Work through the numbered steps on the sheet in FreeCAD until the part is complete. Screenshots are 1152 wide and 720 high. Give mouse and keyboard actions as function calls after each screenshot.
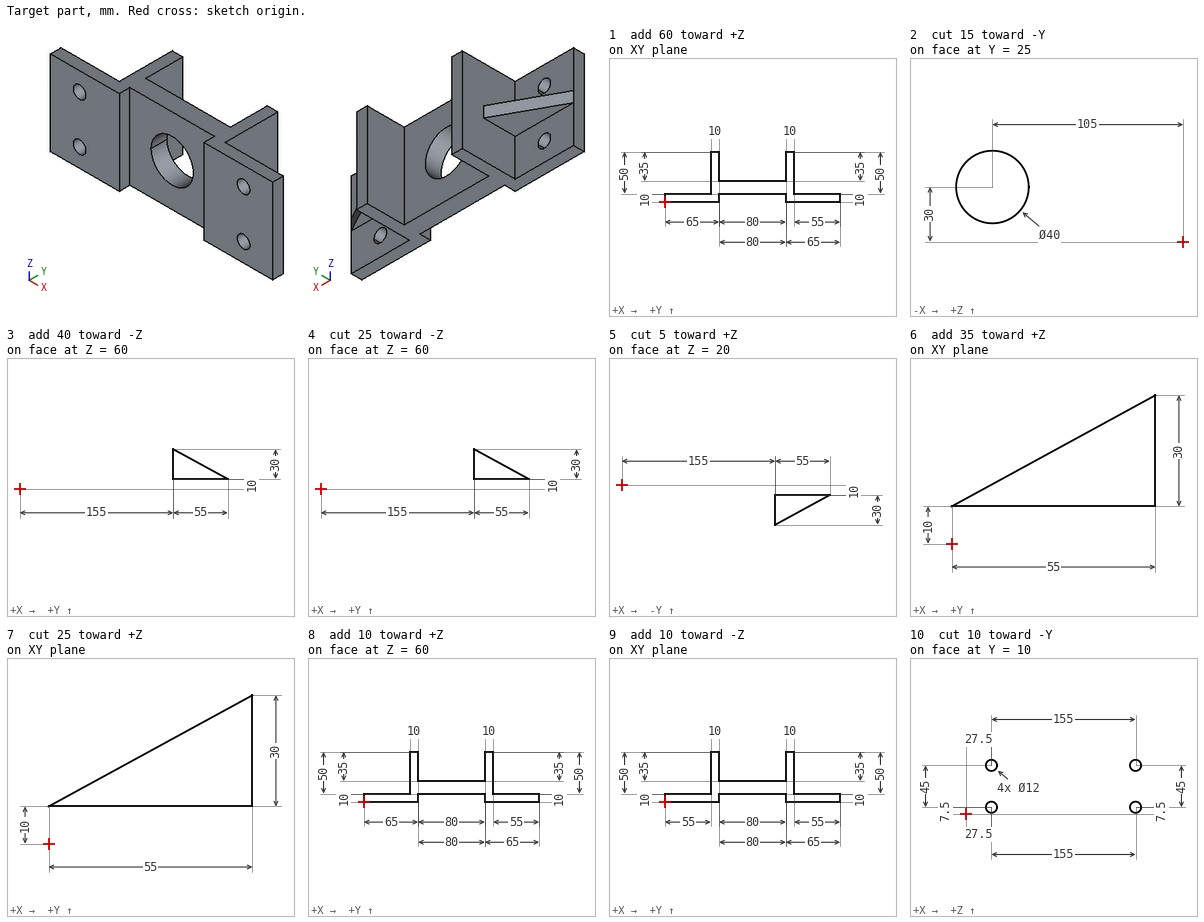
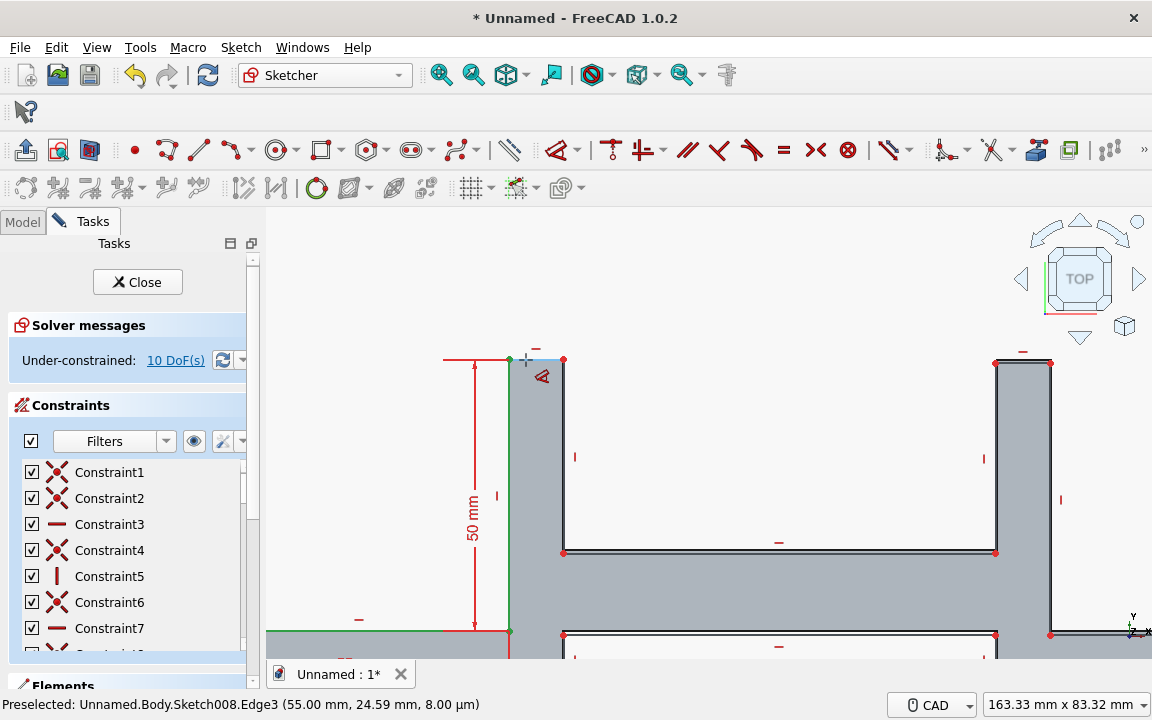
click(525, 360)
click(536, 326)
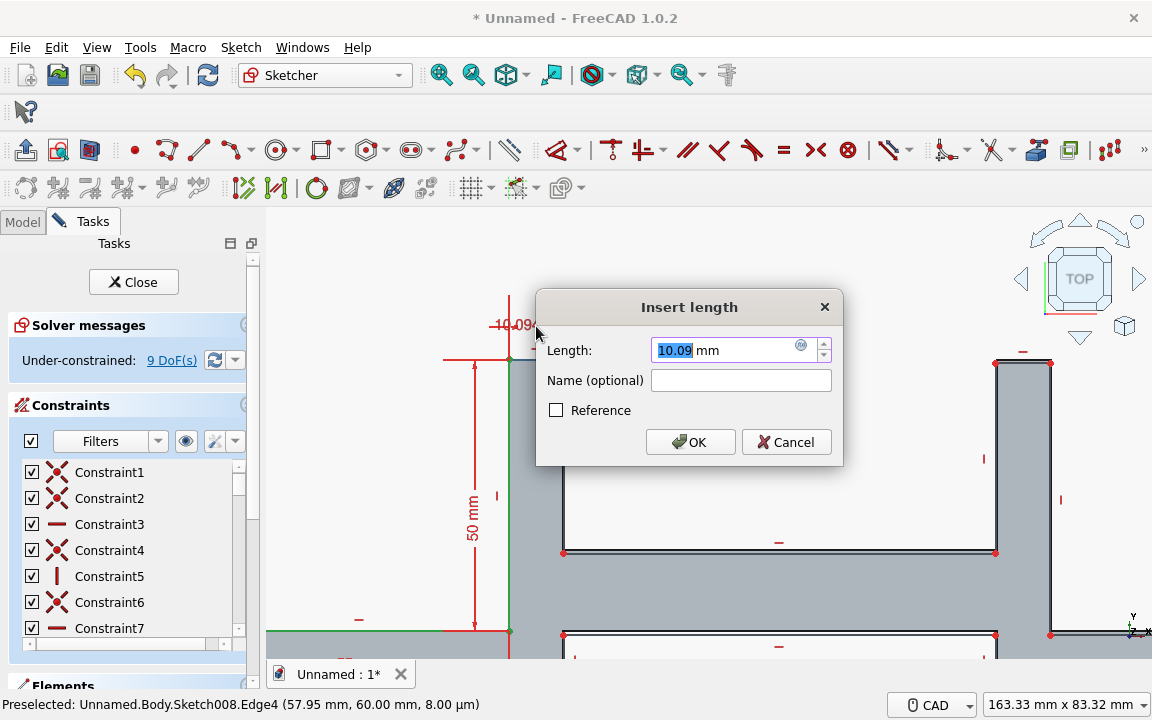
text(10)
key(Return)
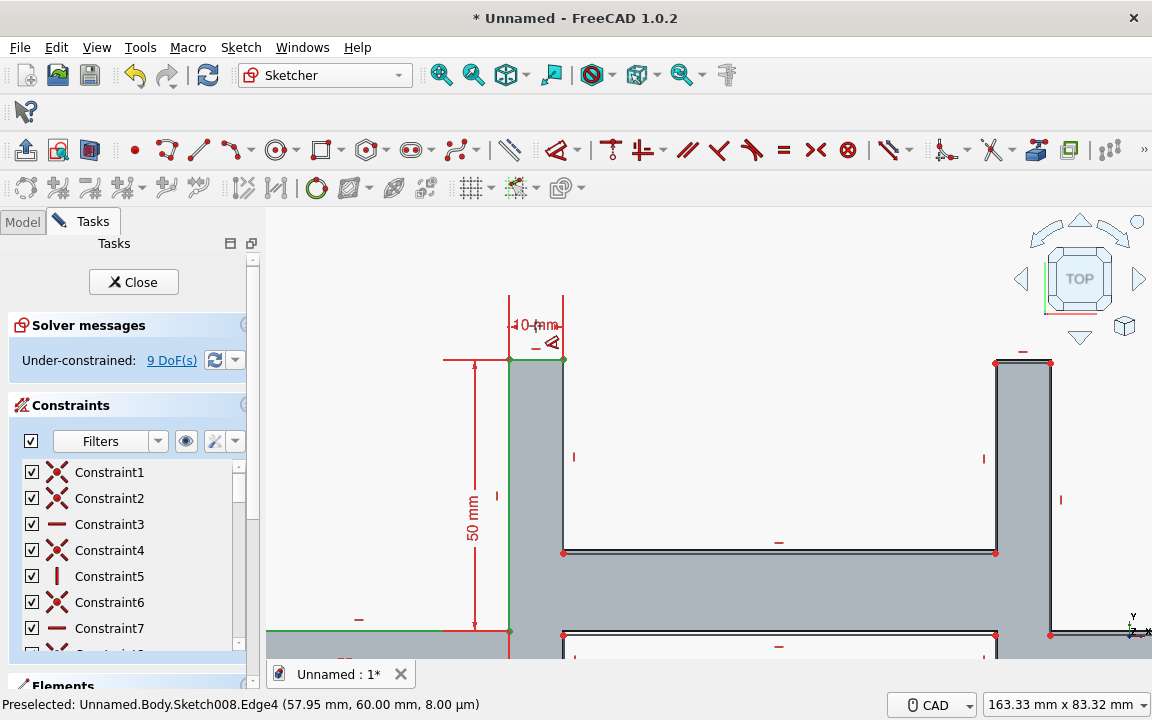
click(563, 418)
click(529, 457)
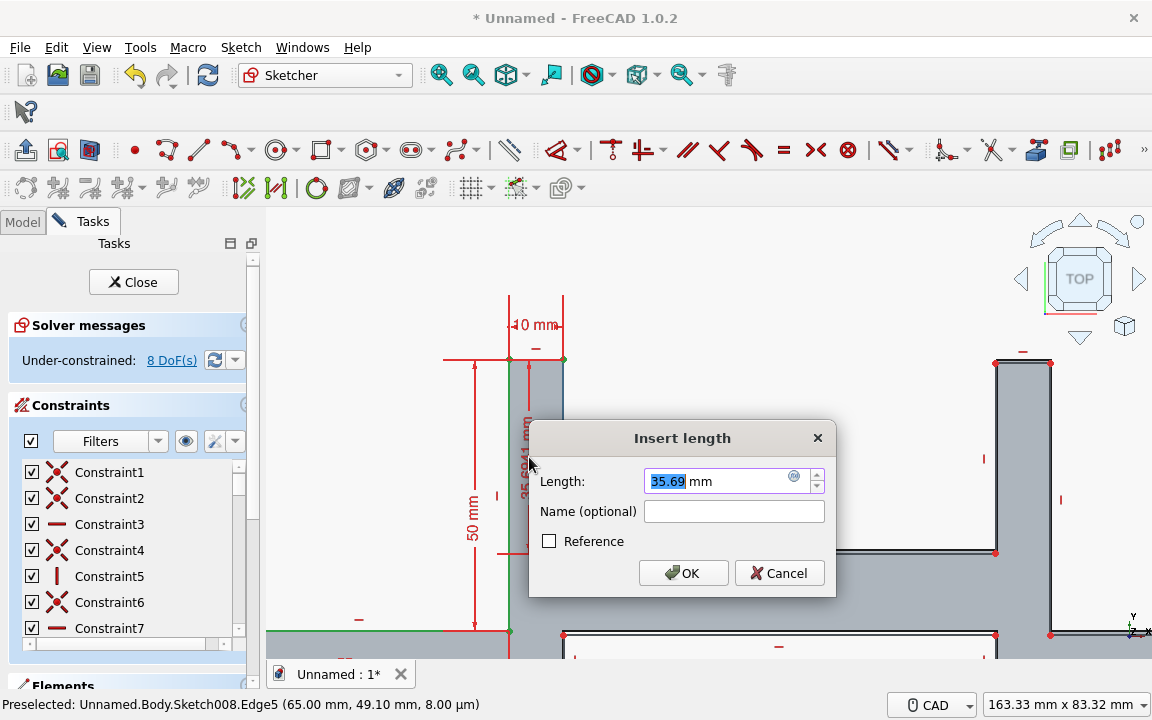
text(35)
key(Return)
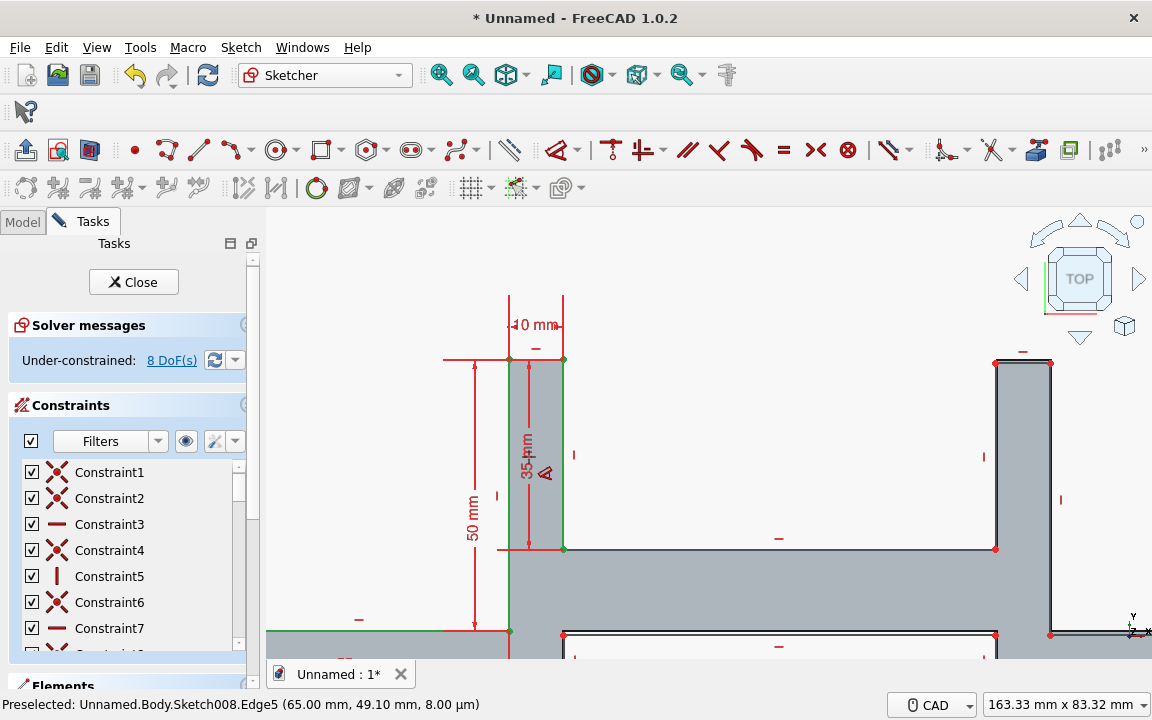
click(693, 550)
click(775, 584)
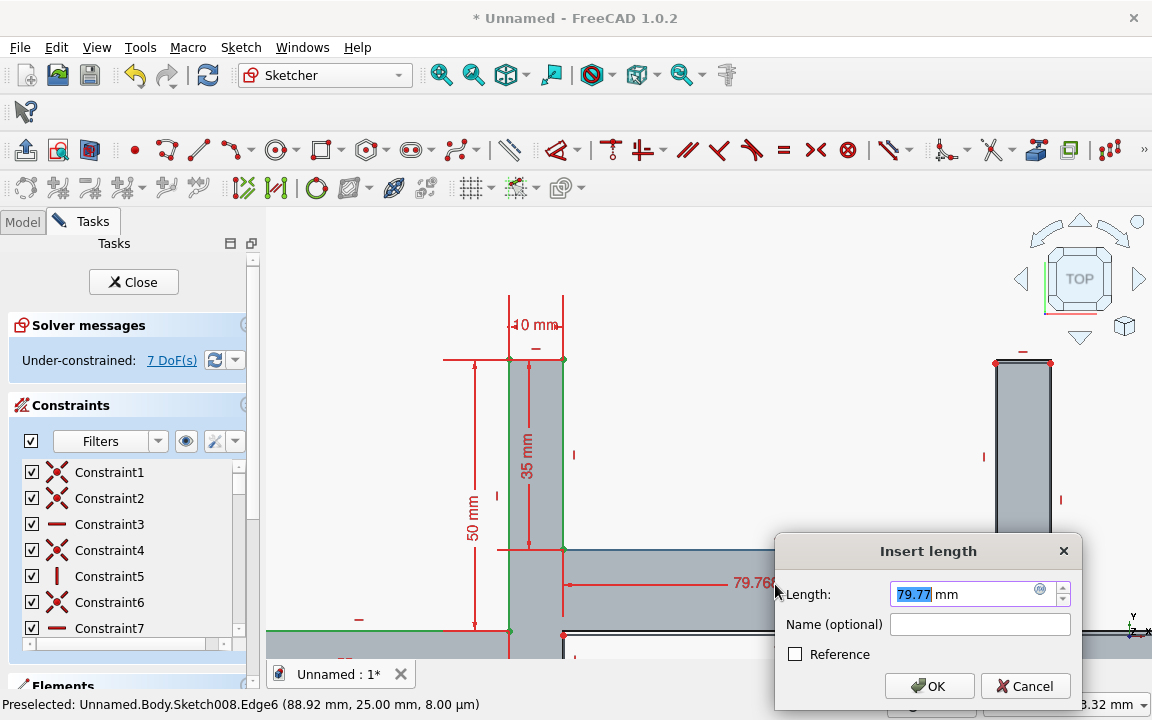
text(80)
key(Return)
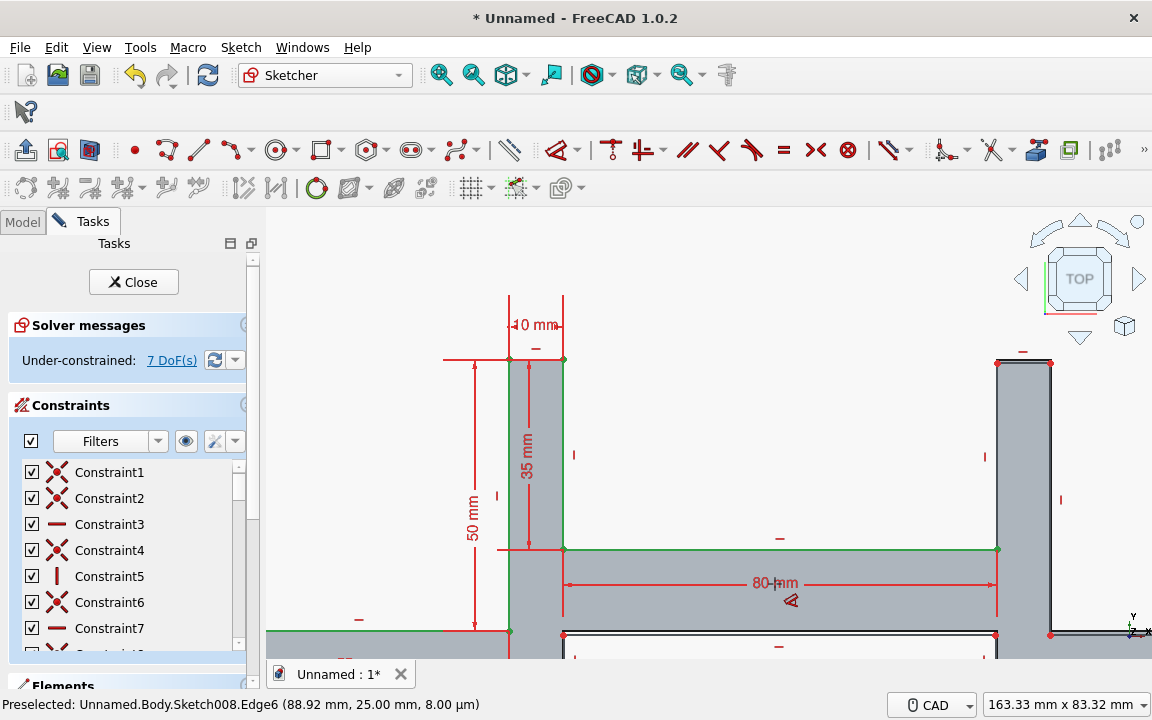
scroll(526, 360, down, 4)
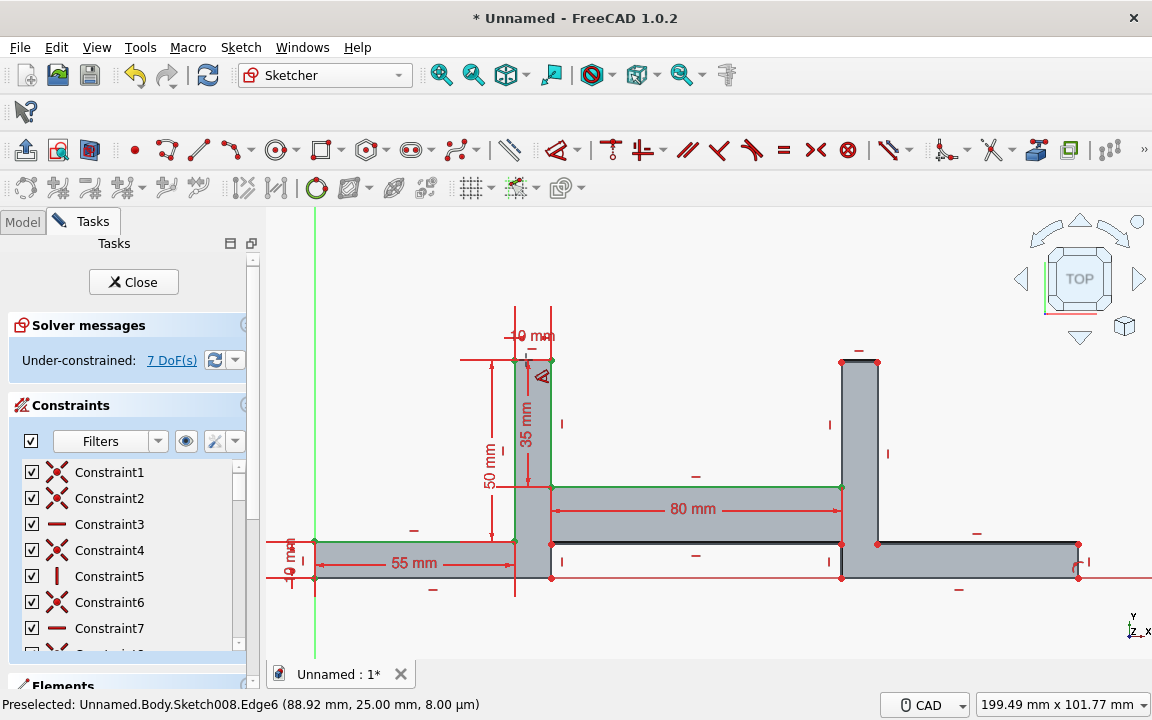
click(738, 420)
click(704, 404)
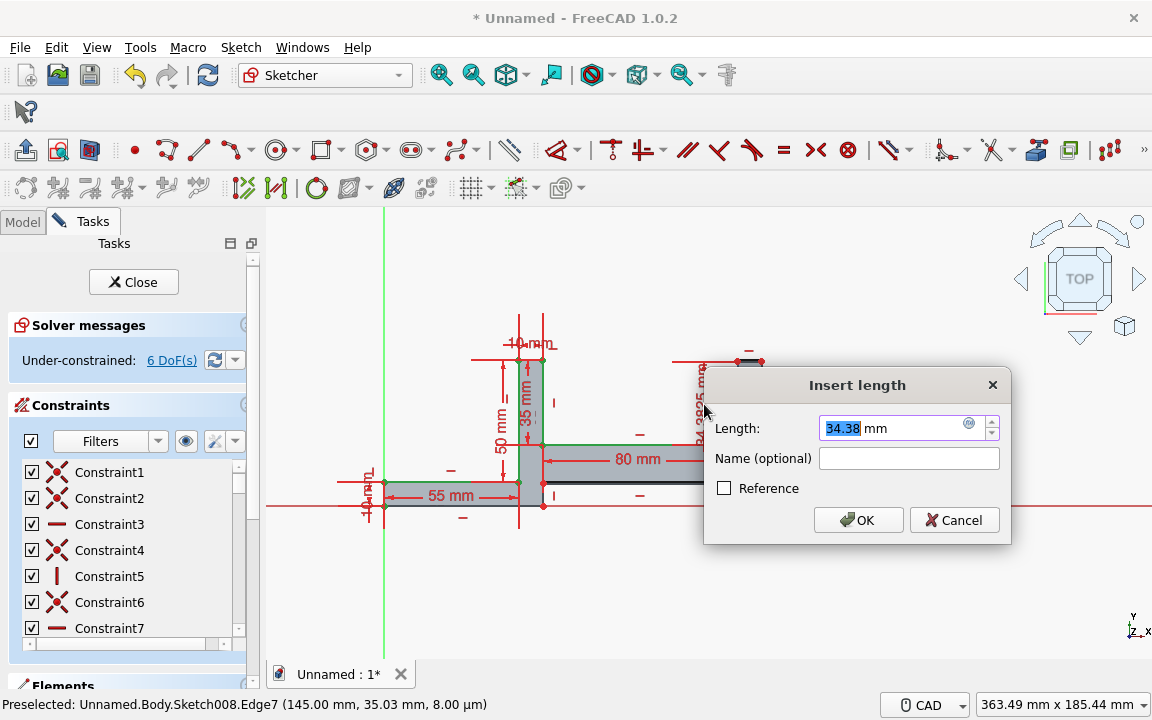
text(35)
key(Return)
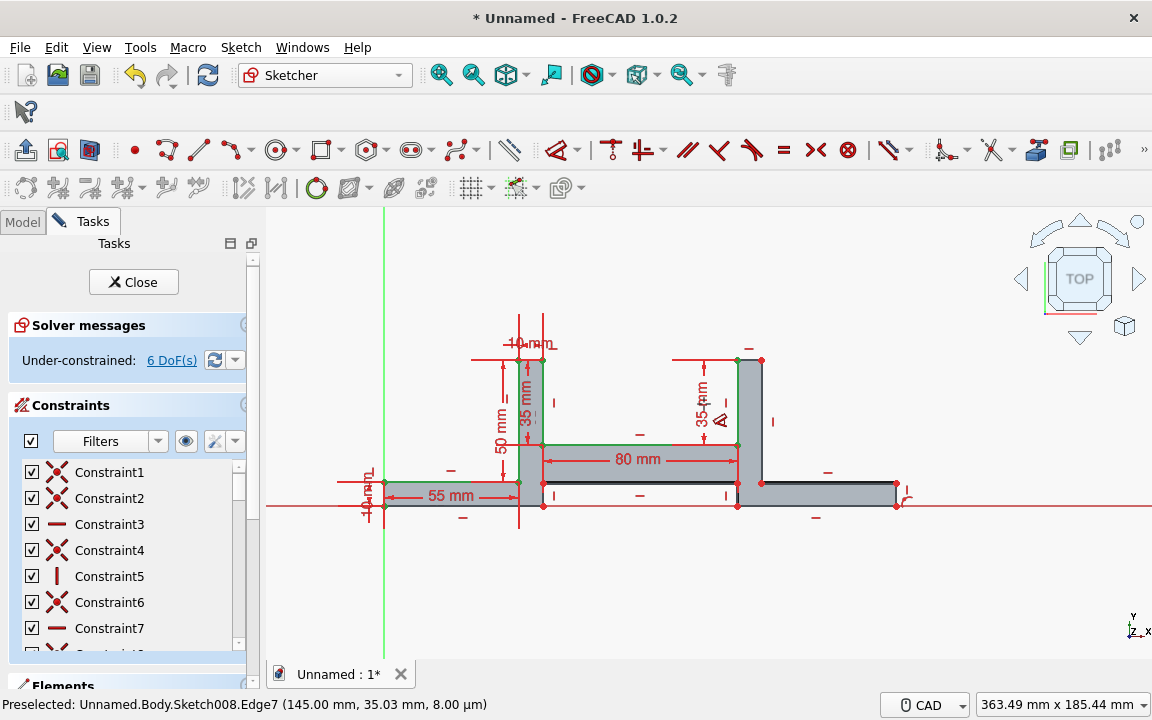
scroll(747, 360, up, 3)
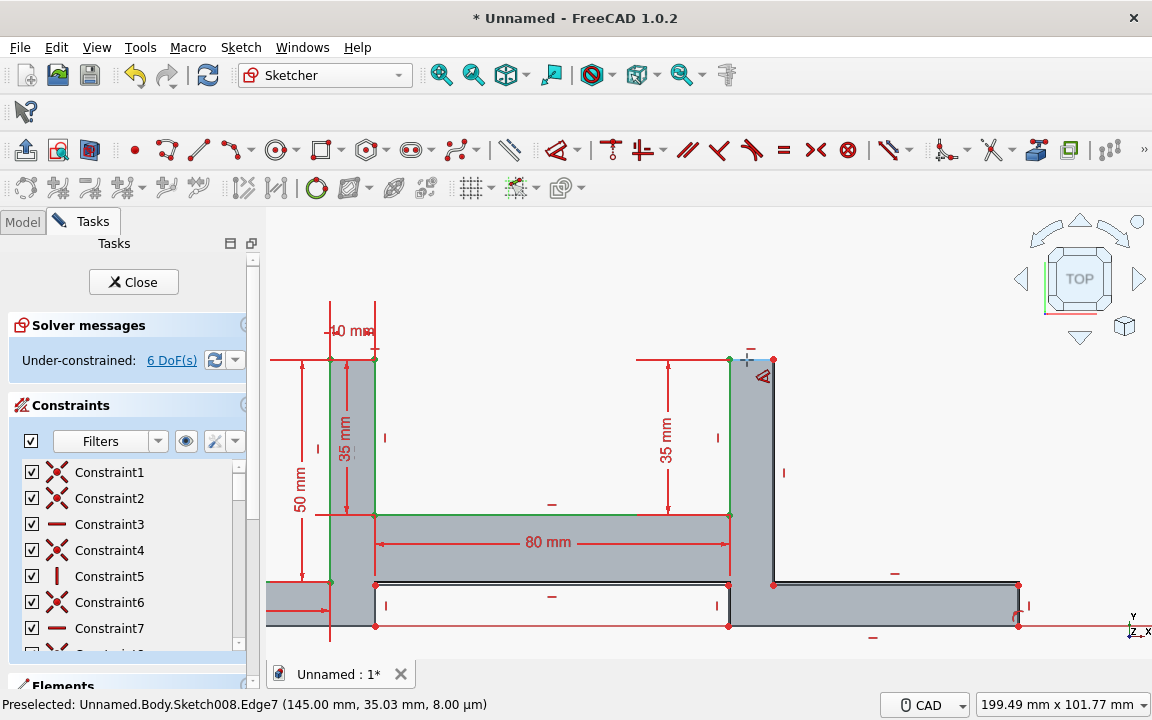
click(747, 360)
click(752, 326)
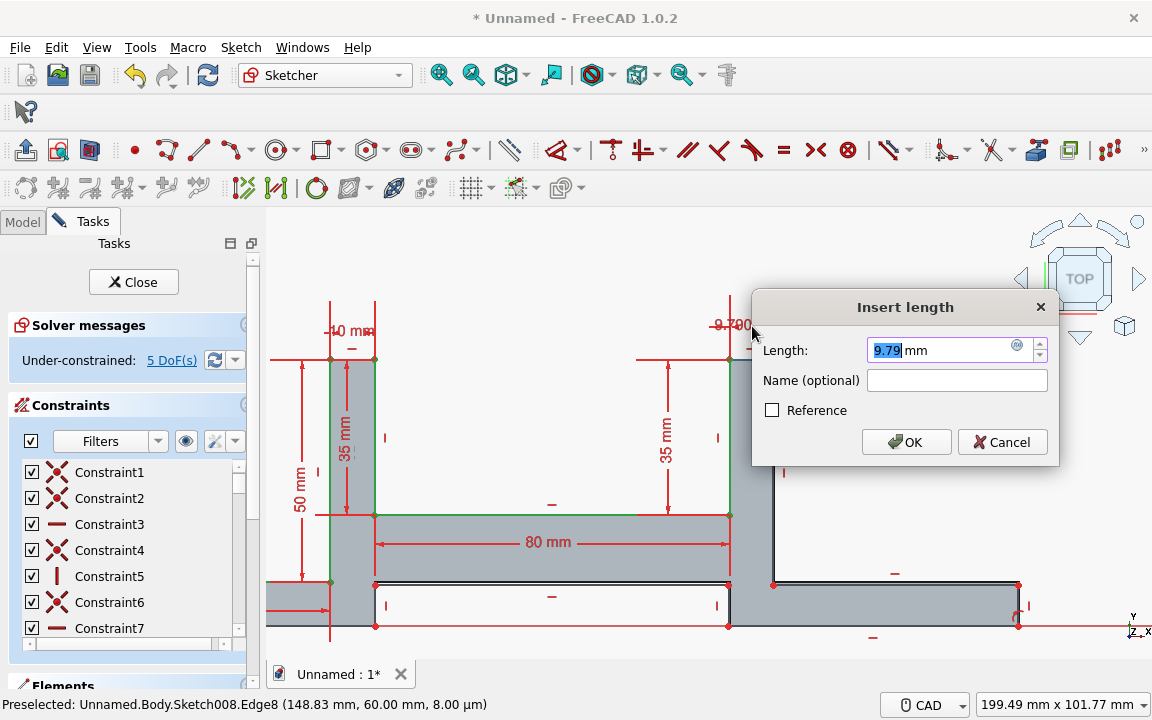
text(10)
key(Return)